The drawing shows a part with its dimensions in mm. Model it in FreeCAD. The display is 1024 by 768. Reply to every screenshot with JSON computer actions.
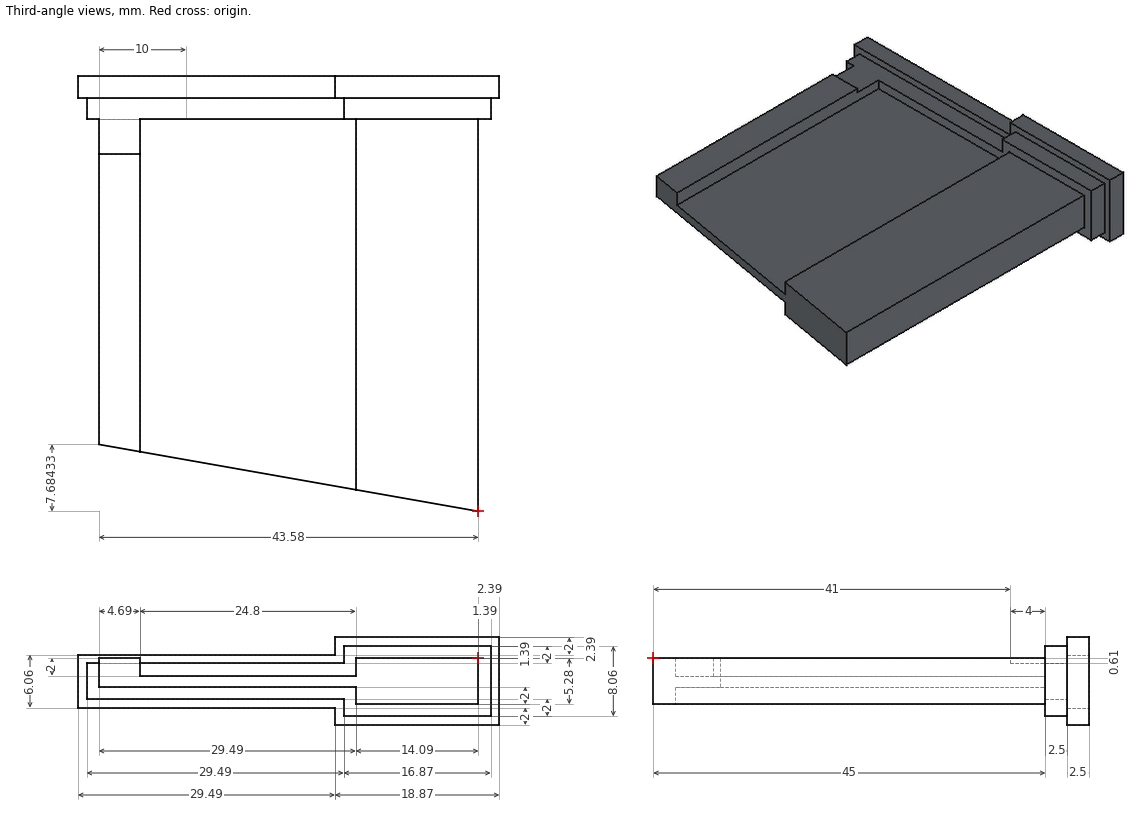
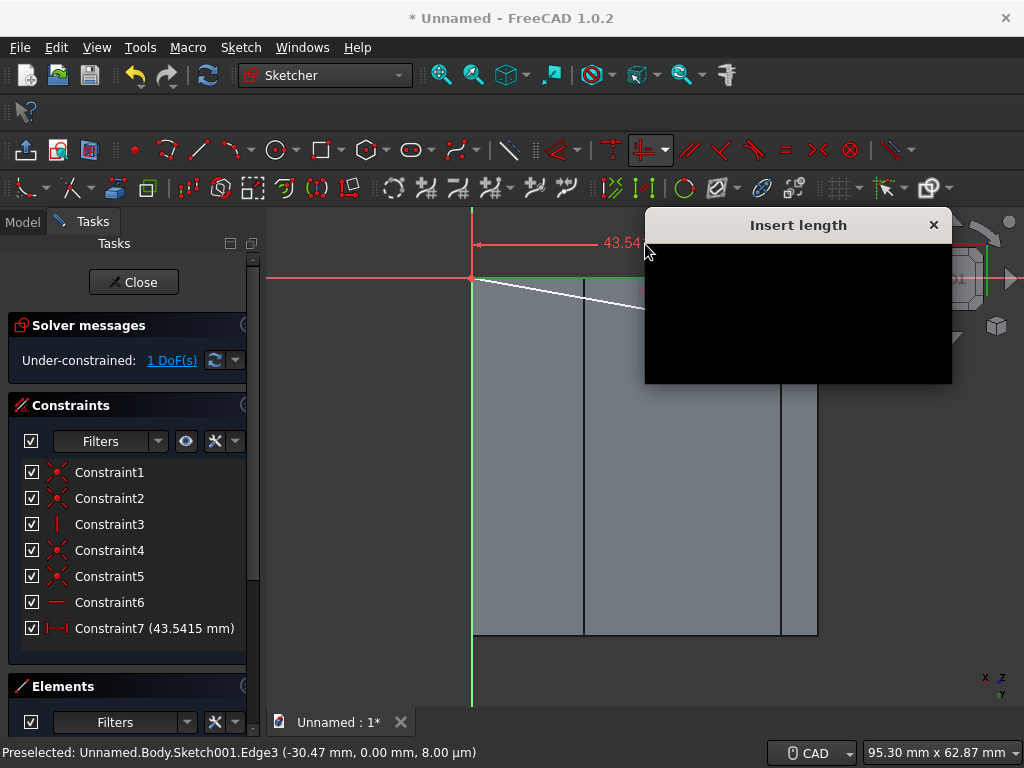
{"action": "type", "text": "43.58"}
{"action": "key", "text": "Return"}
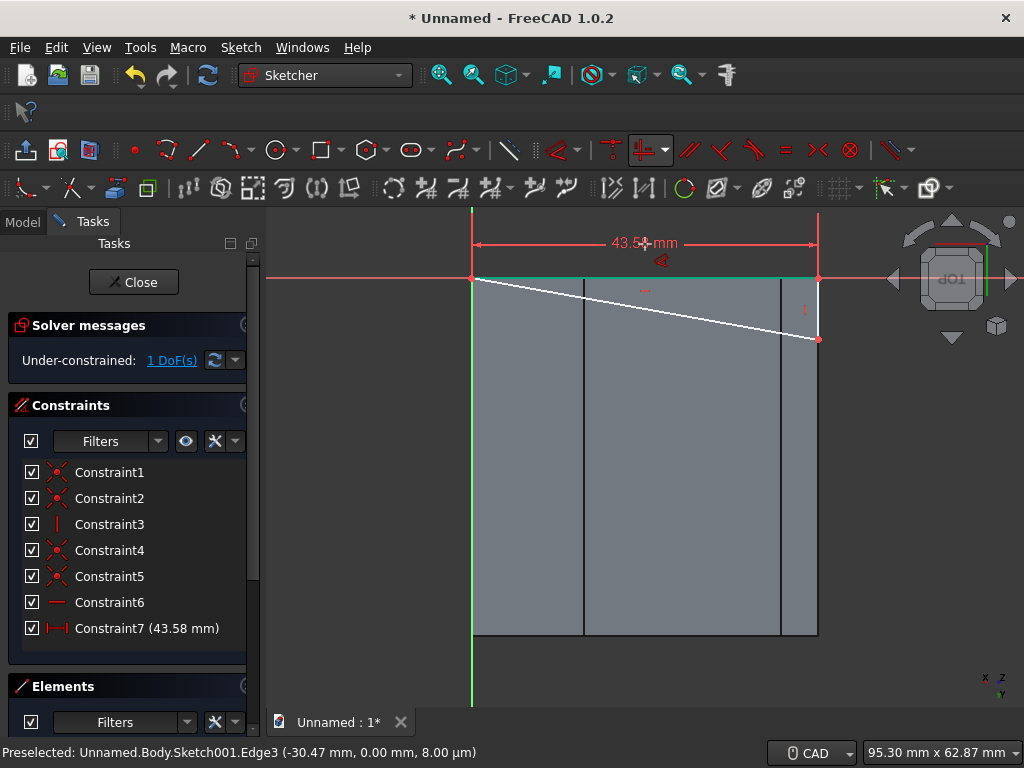
{"action": "left_click", "coordinate": [818, 321]}
{"action": "left_click", "coordinate": [852, 309]}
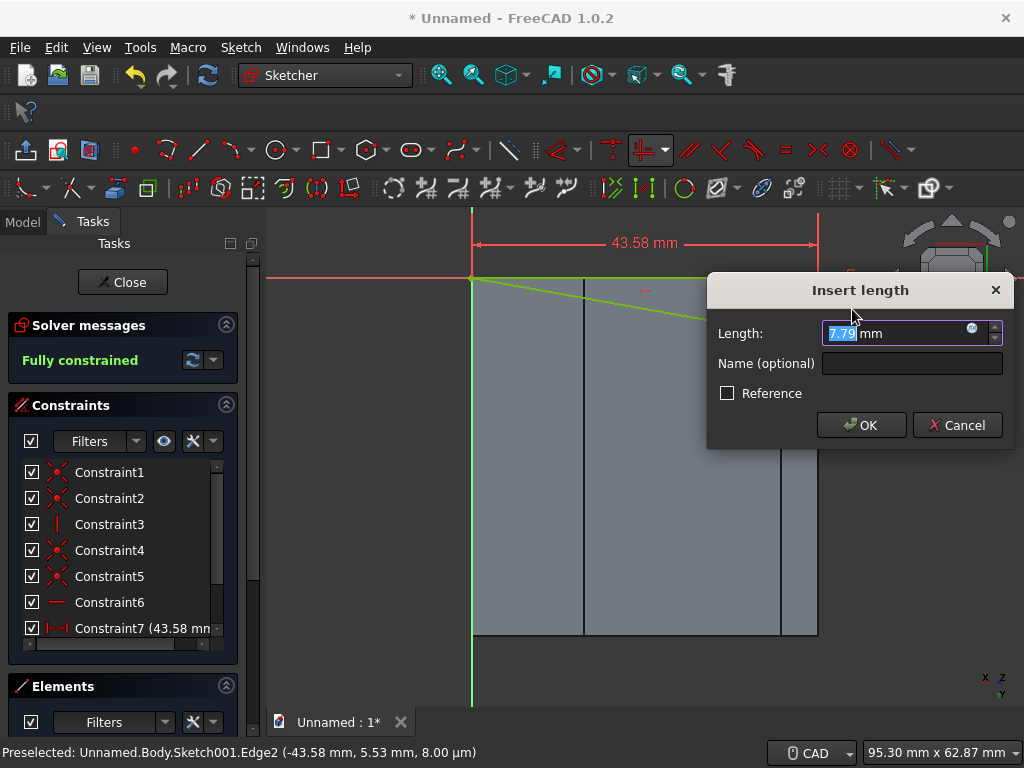
{"action": "type", "text": "7.68433"}
{"action": "key", "text": "Return"}
{"action": "key", "text": "Escape"}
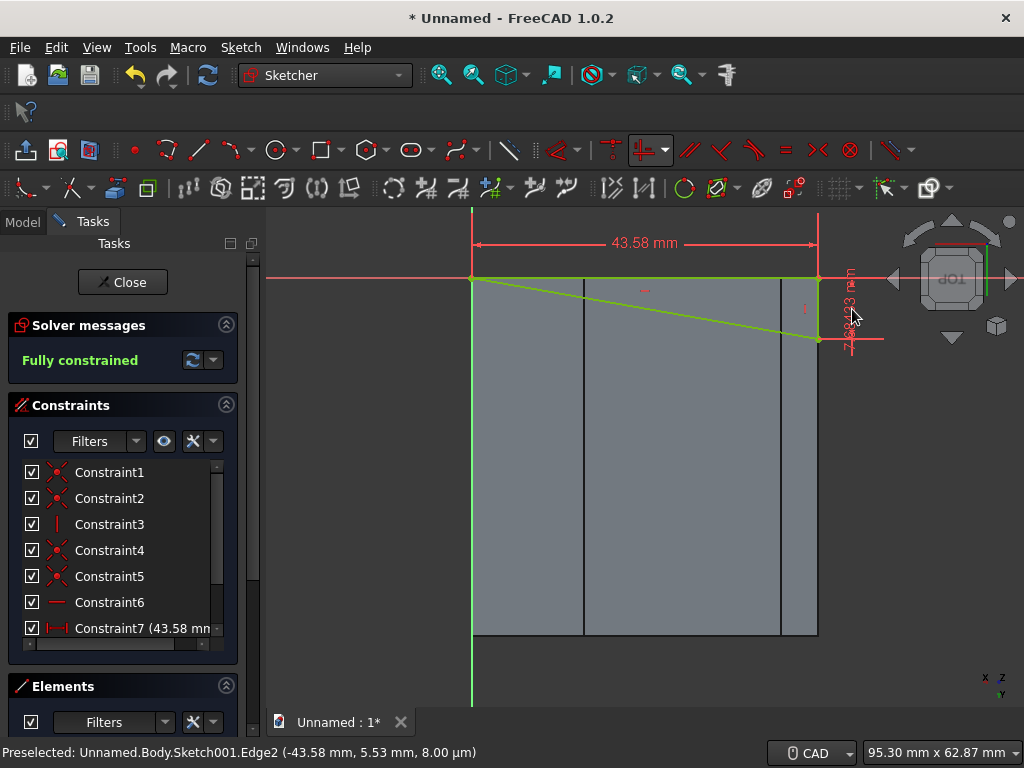
{"action": "left_click", "coordinate": [123, 282]}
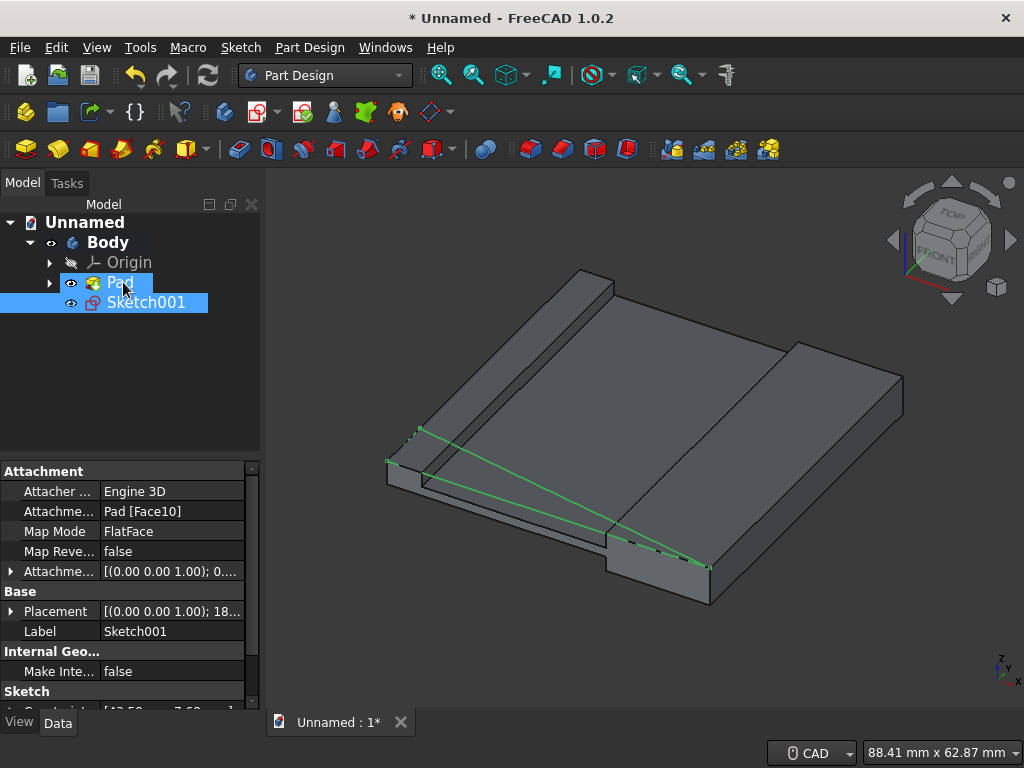
{"action": "left_click", "coordinate": [240, 150]}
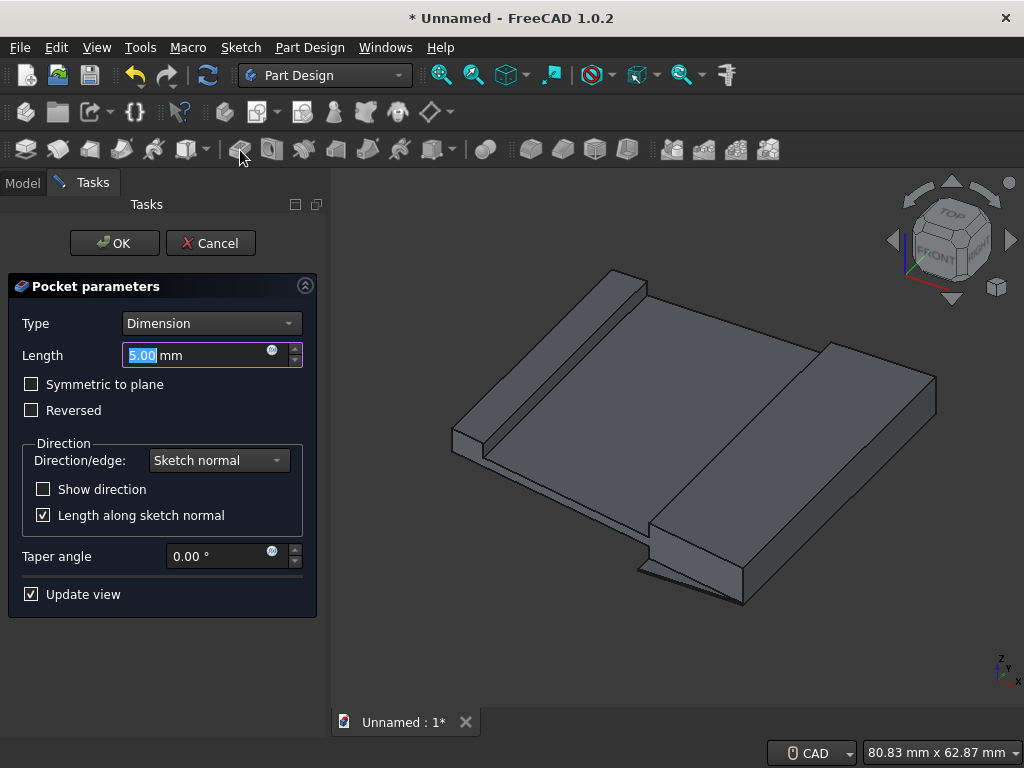
{"action": "left_click", "coordinate": [212, 324]}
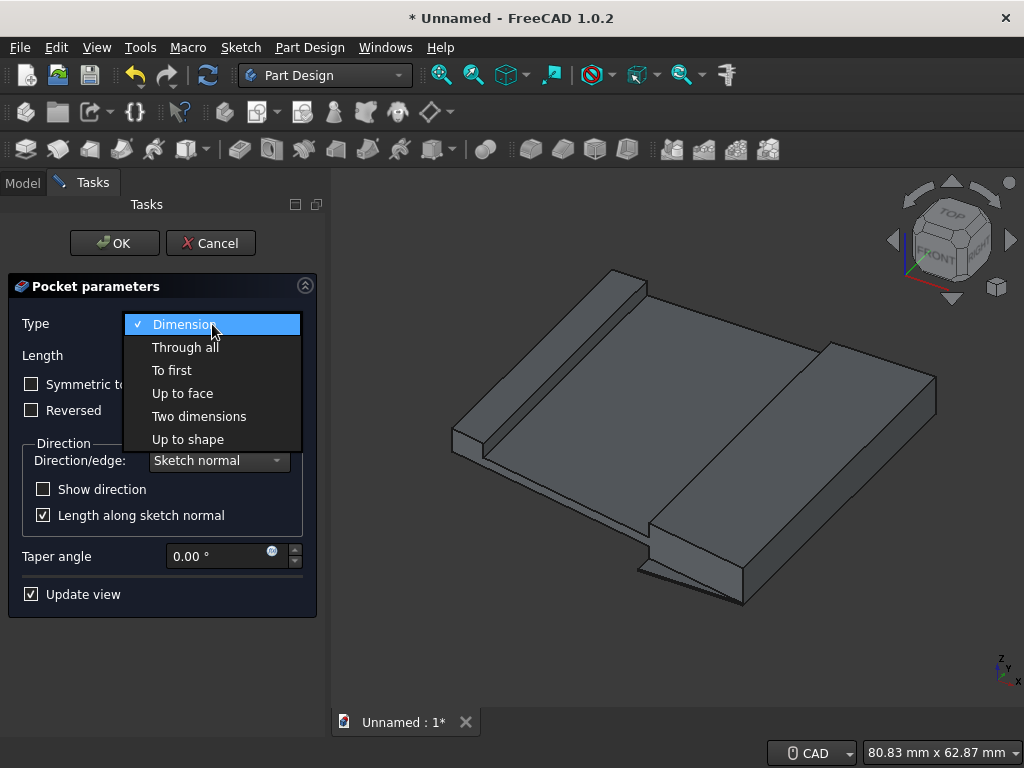
{"action": "left_click", "coordinate": [212, 348]}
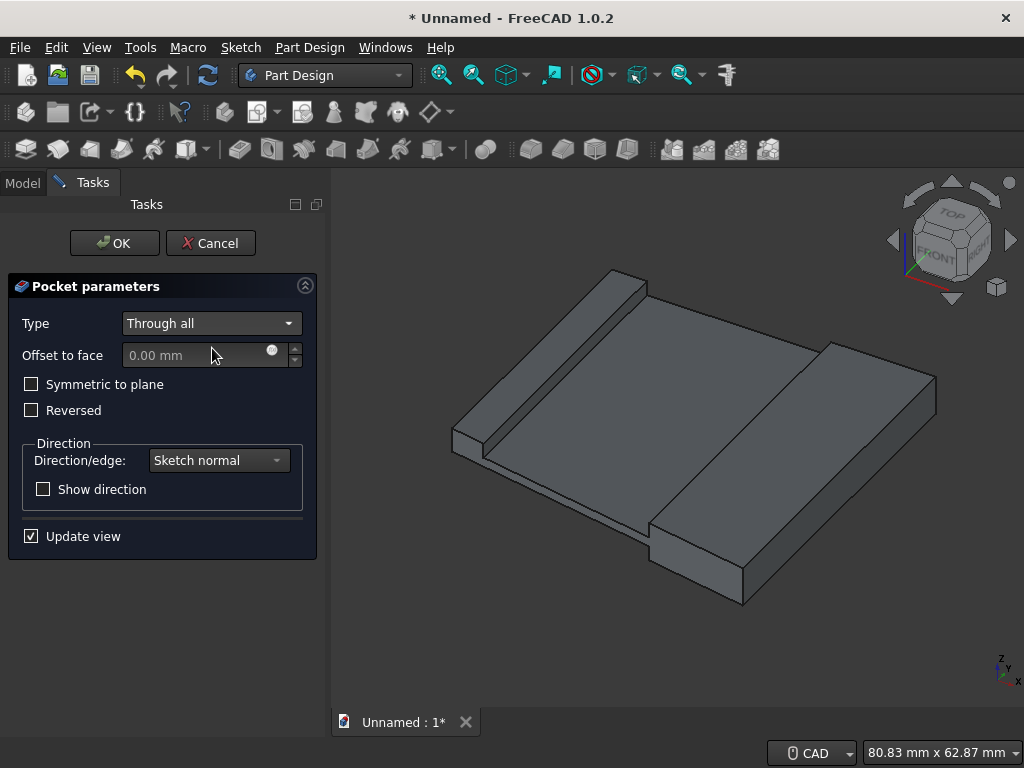
{"action": "left_click", "coordinate": [115, 243]}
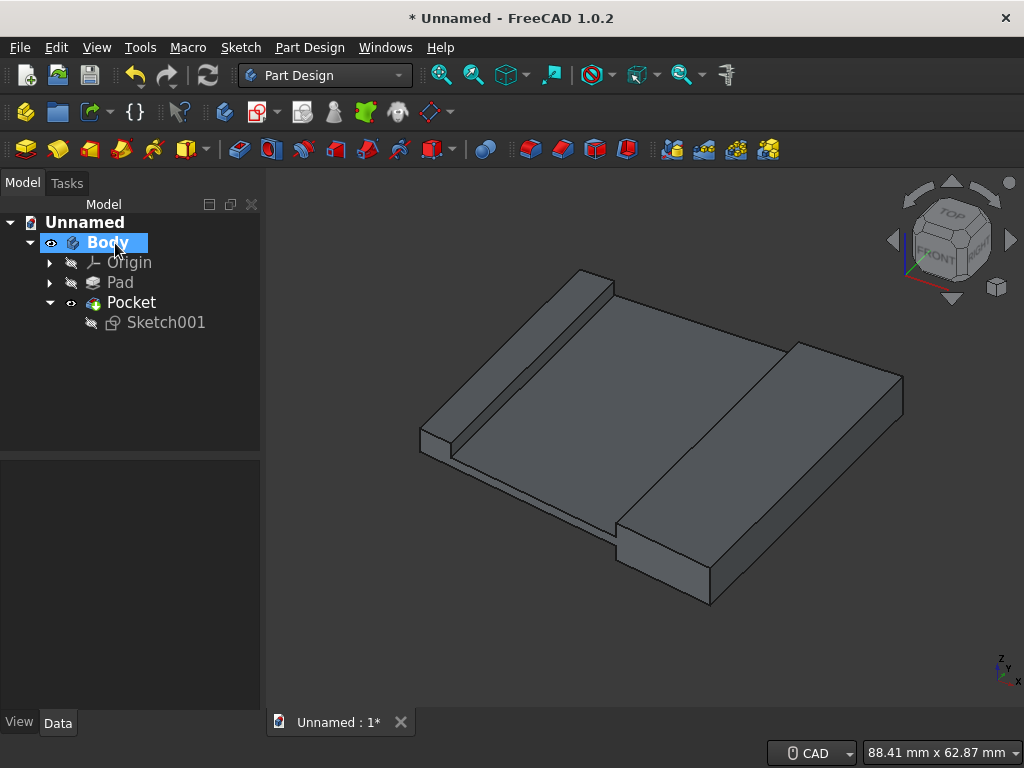
{"action": "key", "text": "4"}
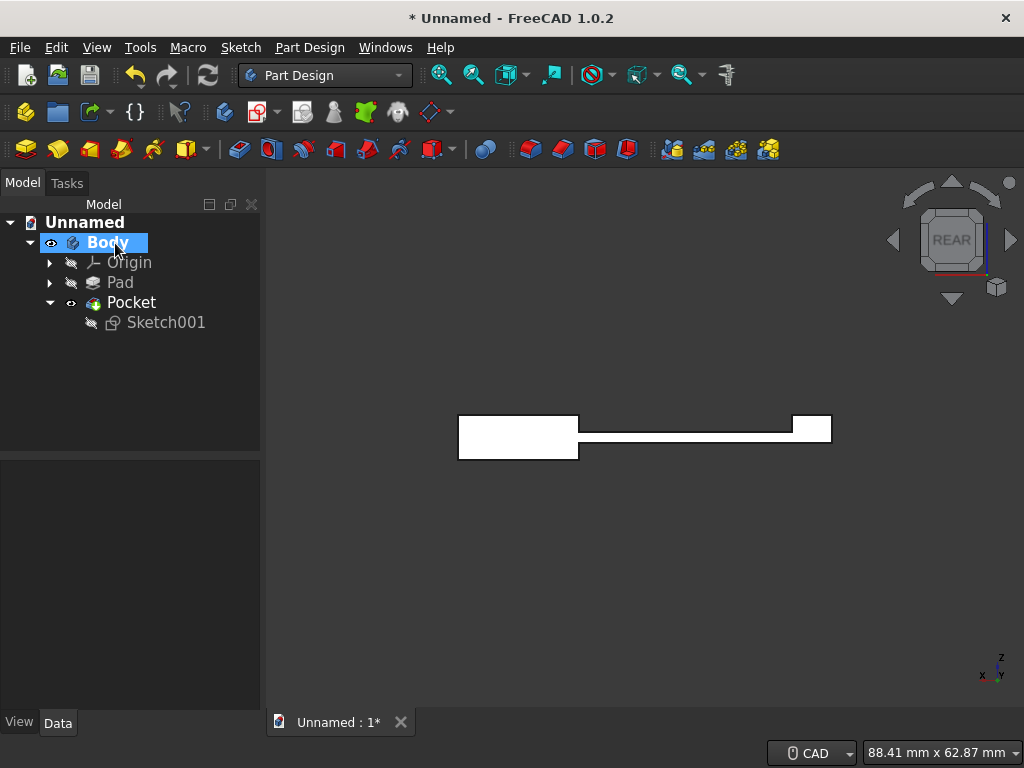
{"action": "left_click", "coordinate": [485, 437]}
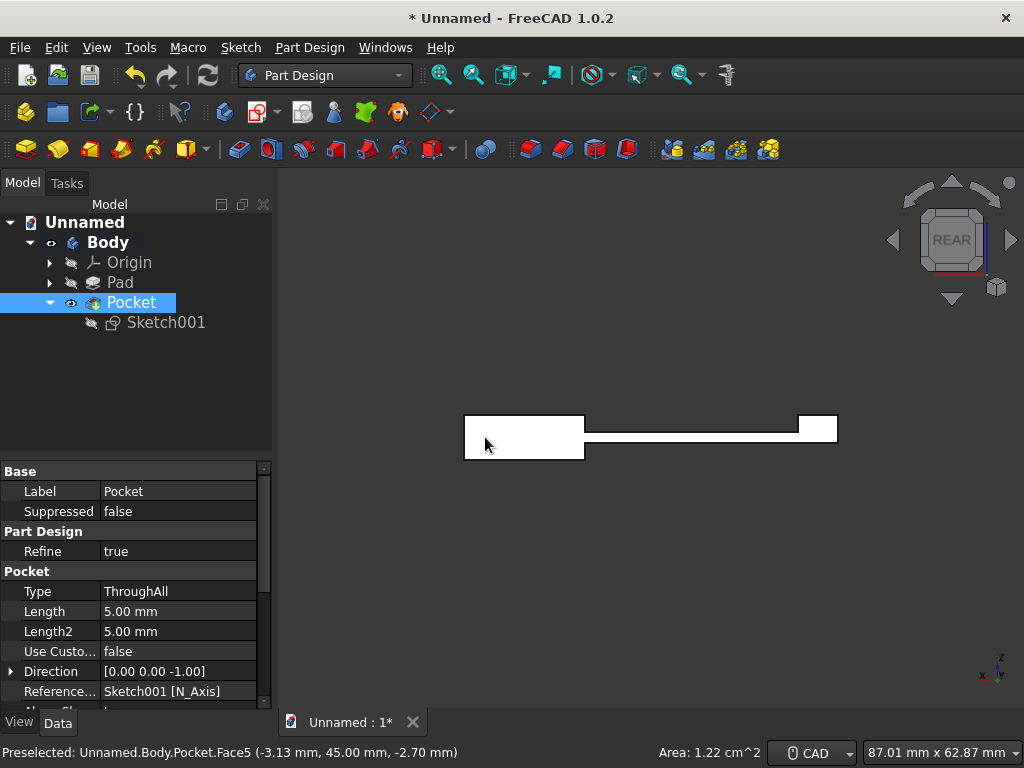
{"action": "left_click", "coordinate": [258, 112]}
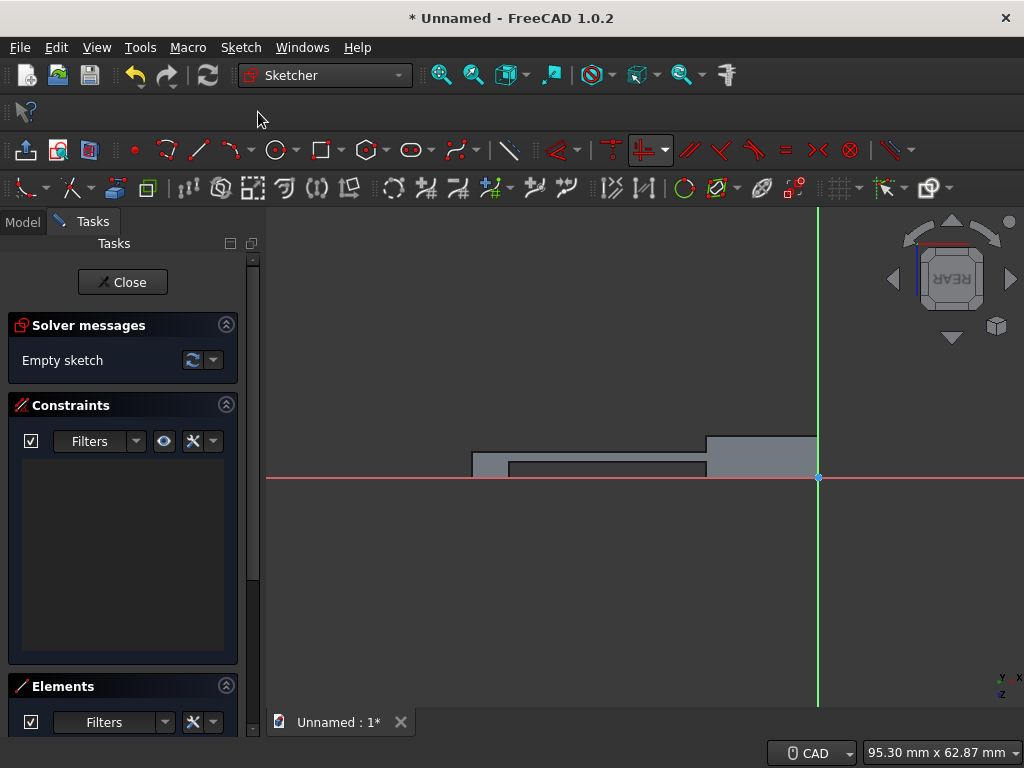
{"action": "key", "text": "g m"}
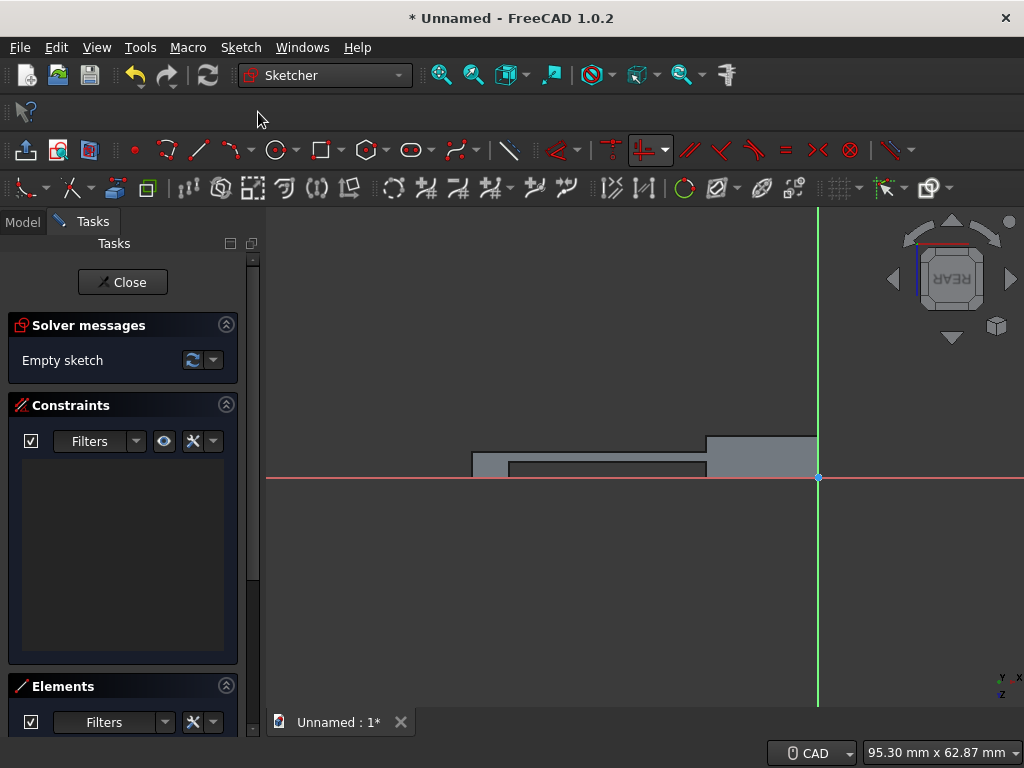
{"action": "scroll", "coordinate": [829, 489], "scroll_direction": "up", "scroll_amount": 2}